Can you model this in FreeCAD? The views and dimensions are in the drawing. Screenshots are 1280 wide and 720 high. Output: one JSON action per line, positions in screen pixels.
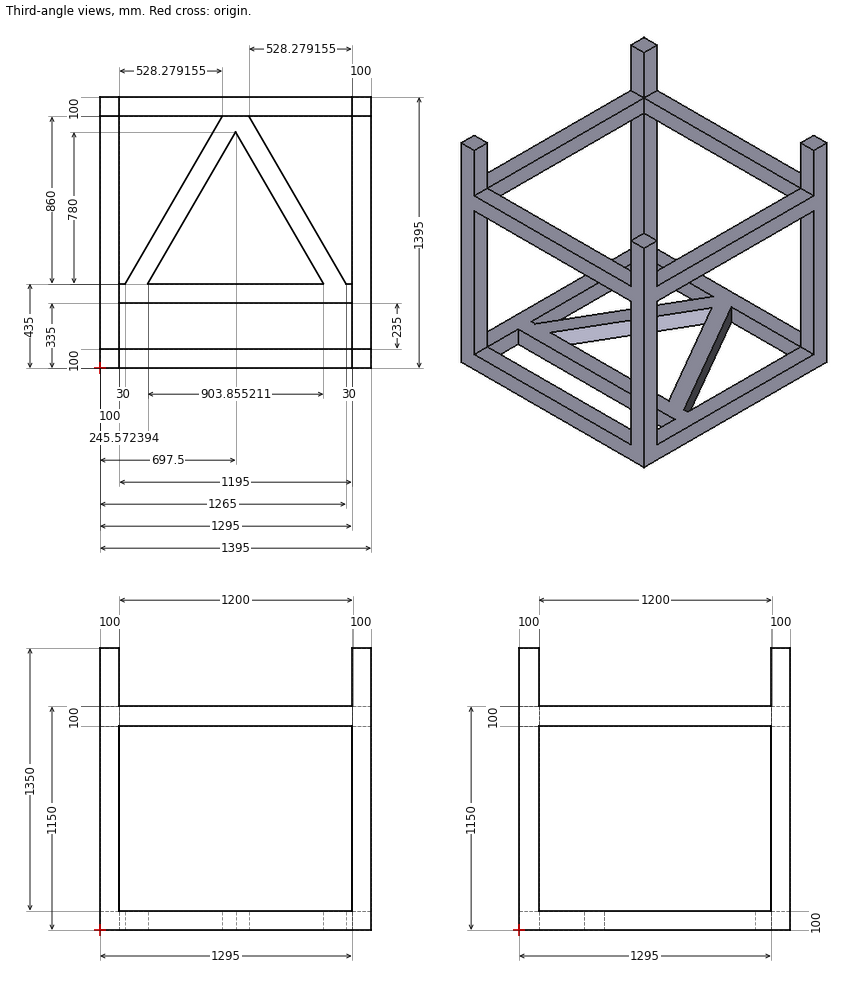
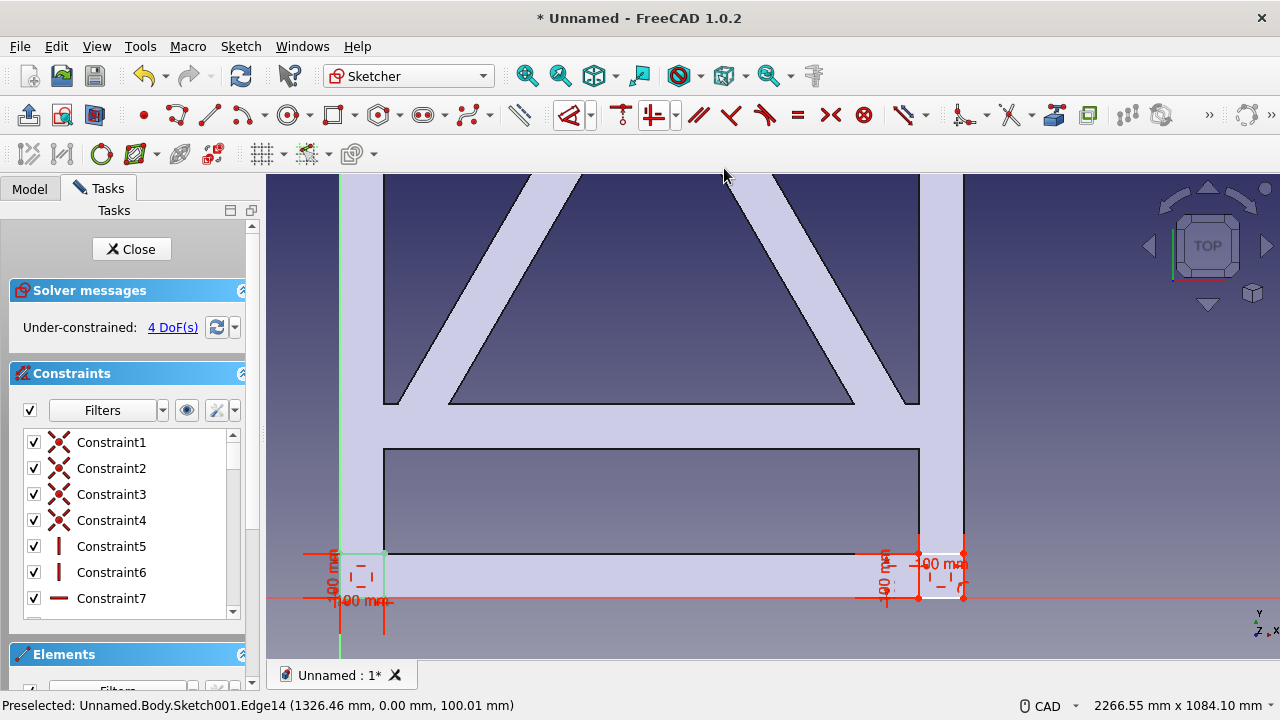
{"action": "scroll", "coordinate": [748, 523], "scroll_direction": "down", "scroll_amount": 4}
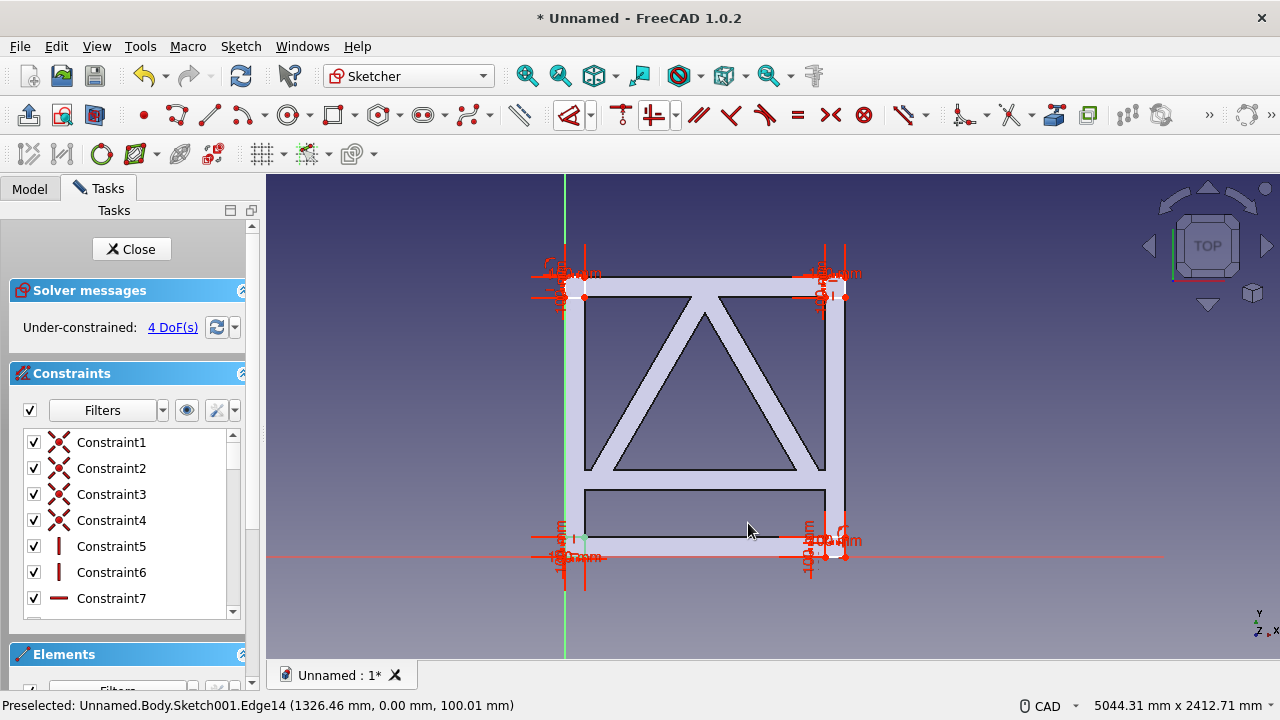
{"action": "left_click", "coordinate": [565, 277]}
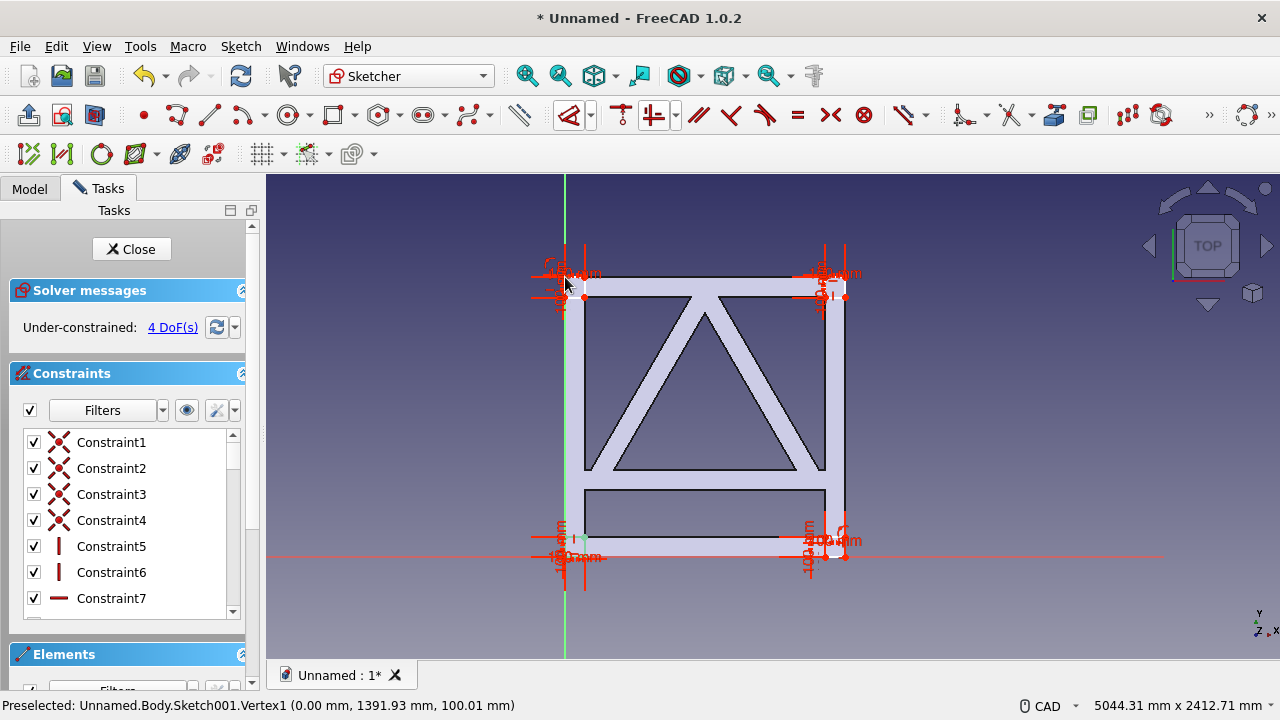
{"action": "left_click", "coordinate": [590, 116]}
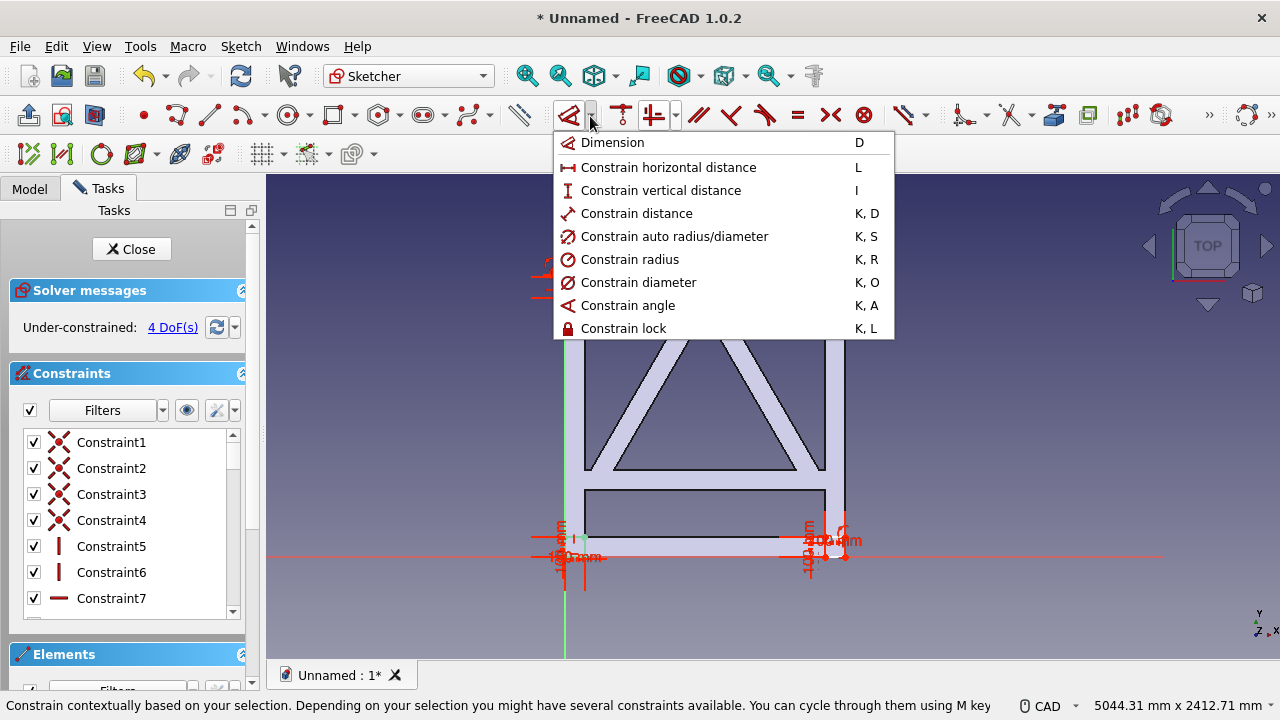
{"action": "left_click", "coordinate": [724, 190]}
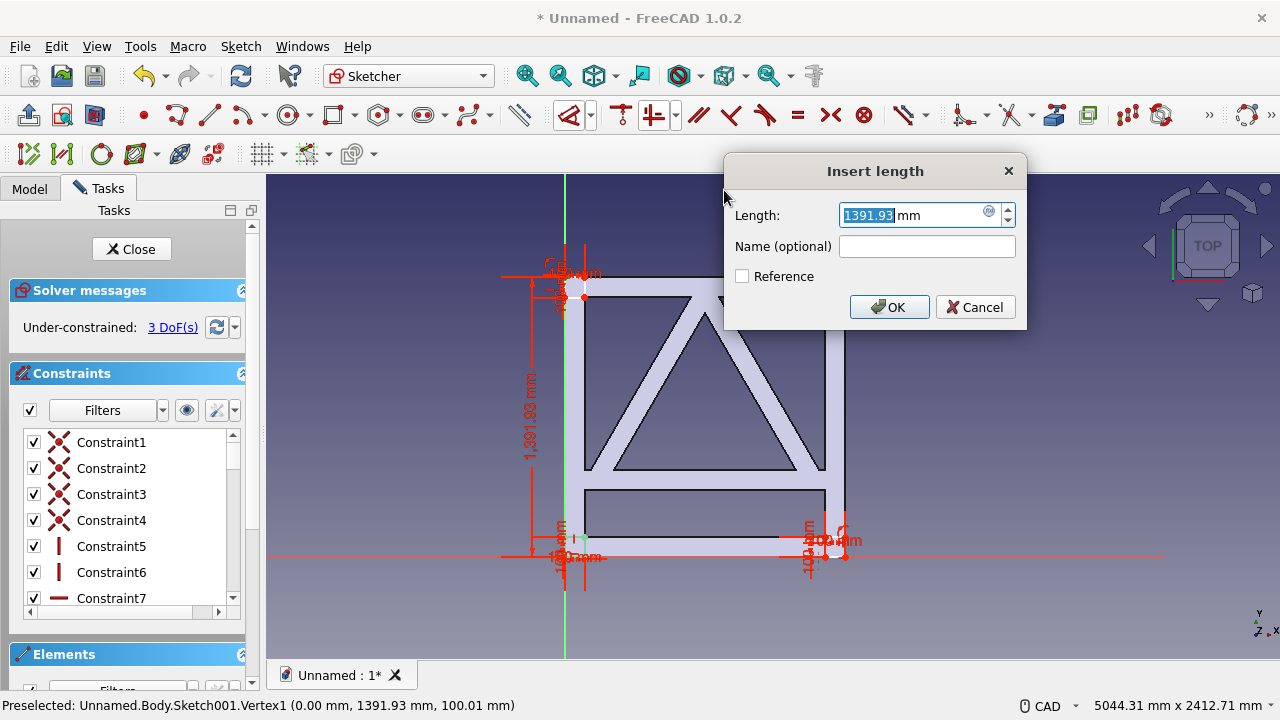
{"action": "type", "text": "1395"}
{"action": "key", "text": "Return"}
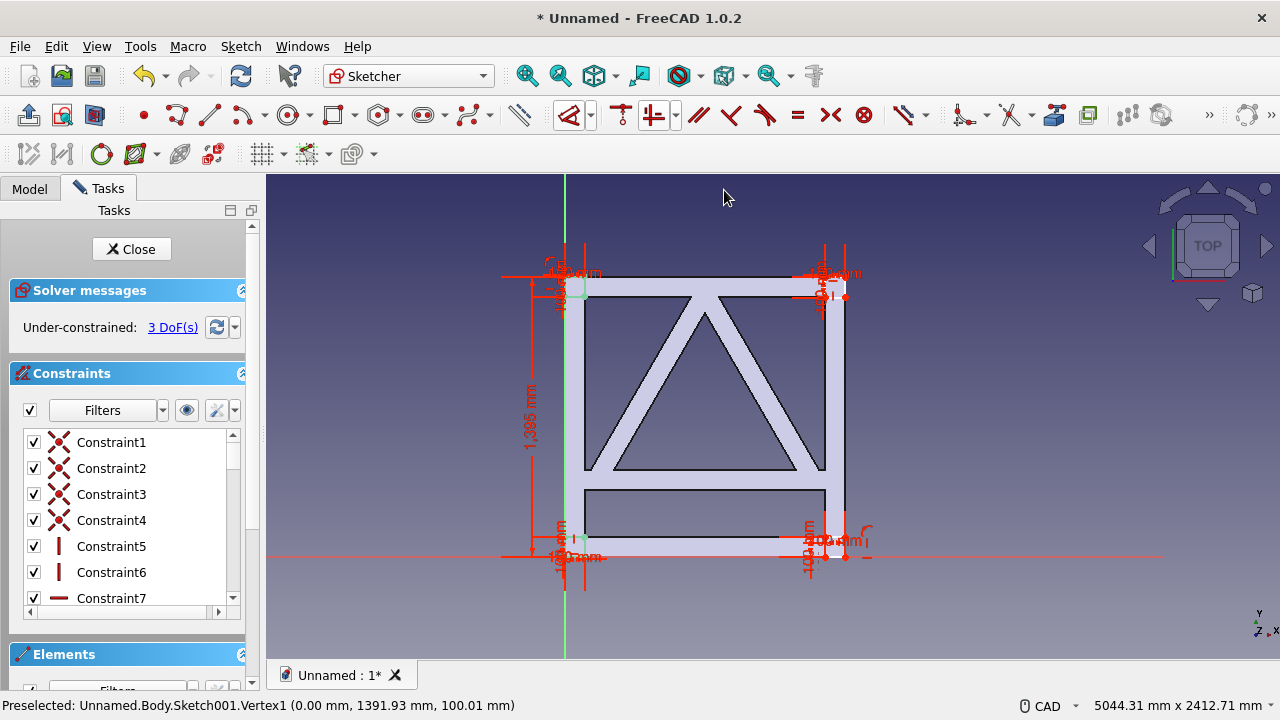
{"action": "left_click", "coordinate": [825, 277]}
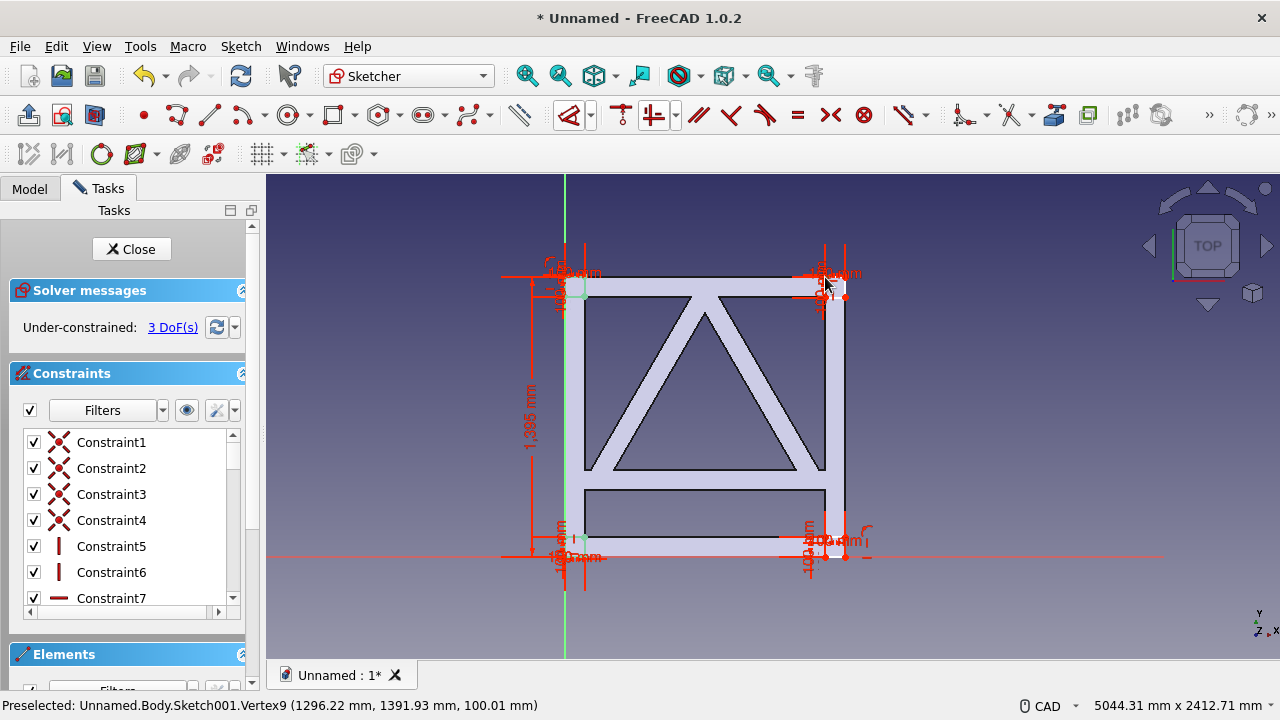
{"action": "left_click", "coordinate": [590, 116]}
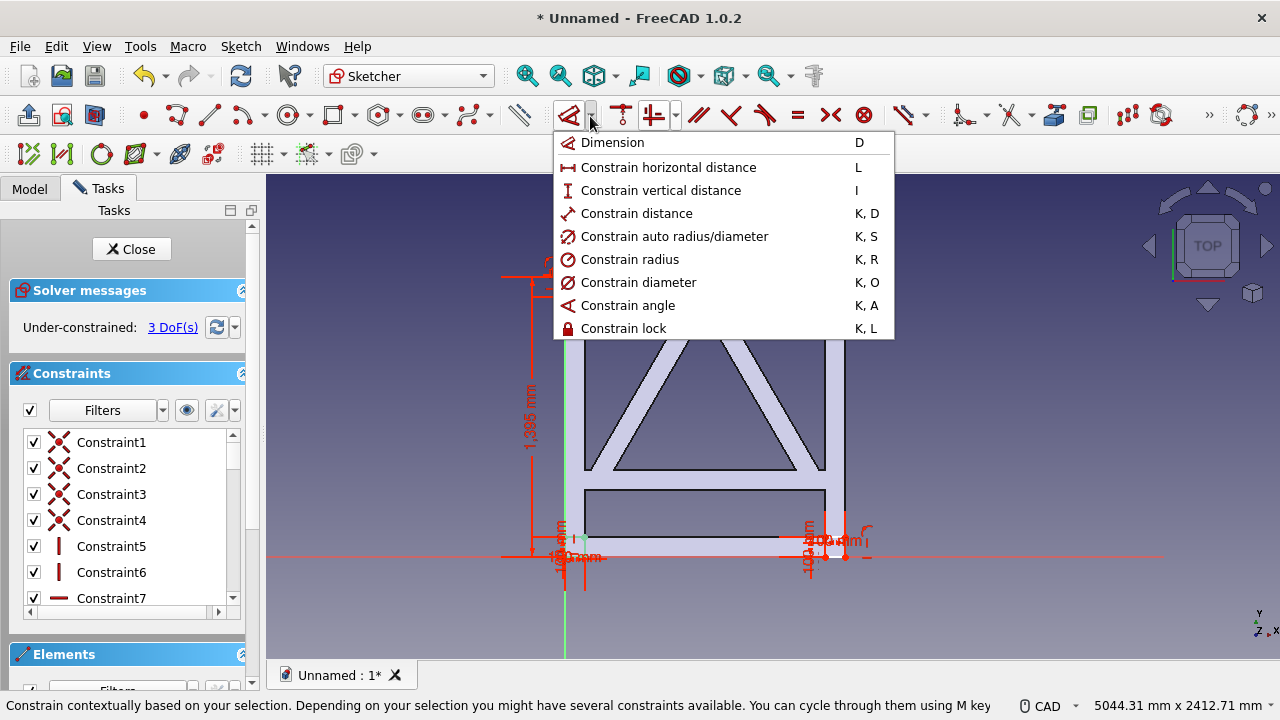
{"action": "left_click", "coordinate": [724, 168]}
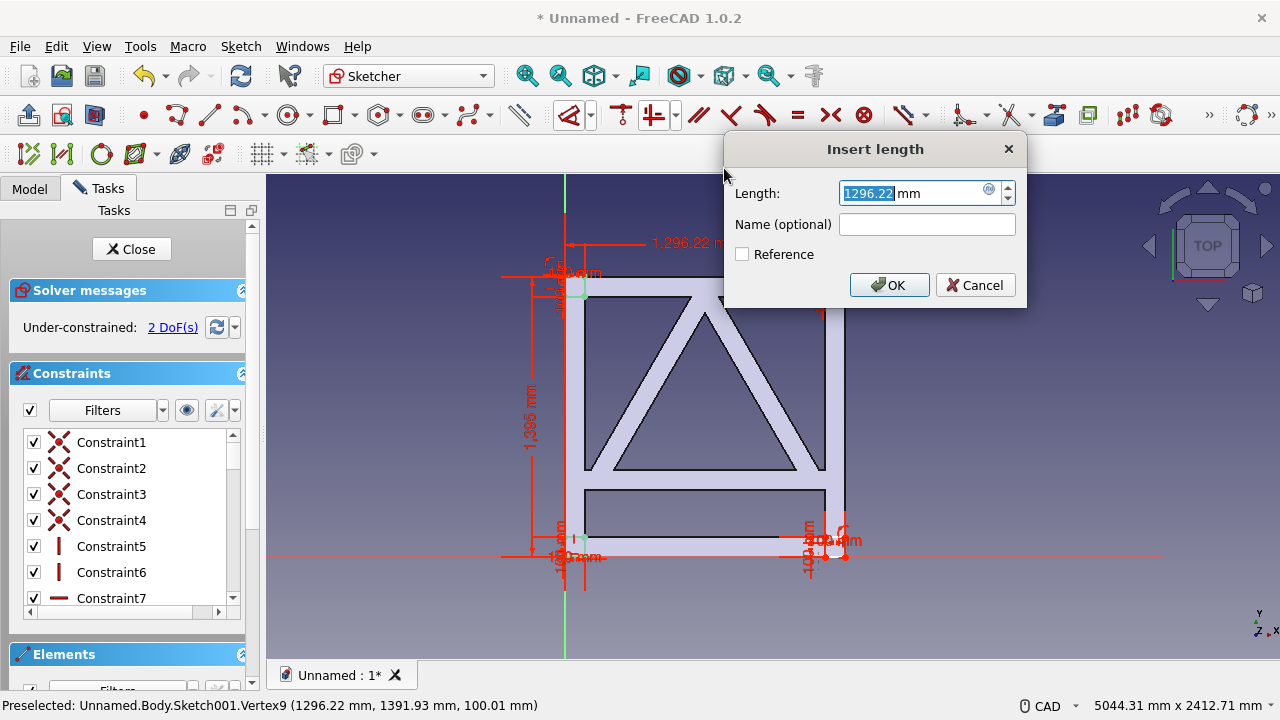
{"action": "type", "text": "1295"}
{"action": "key", "text": "Return"}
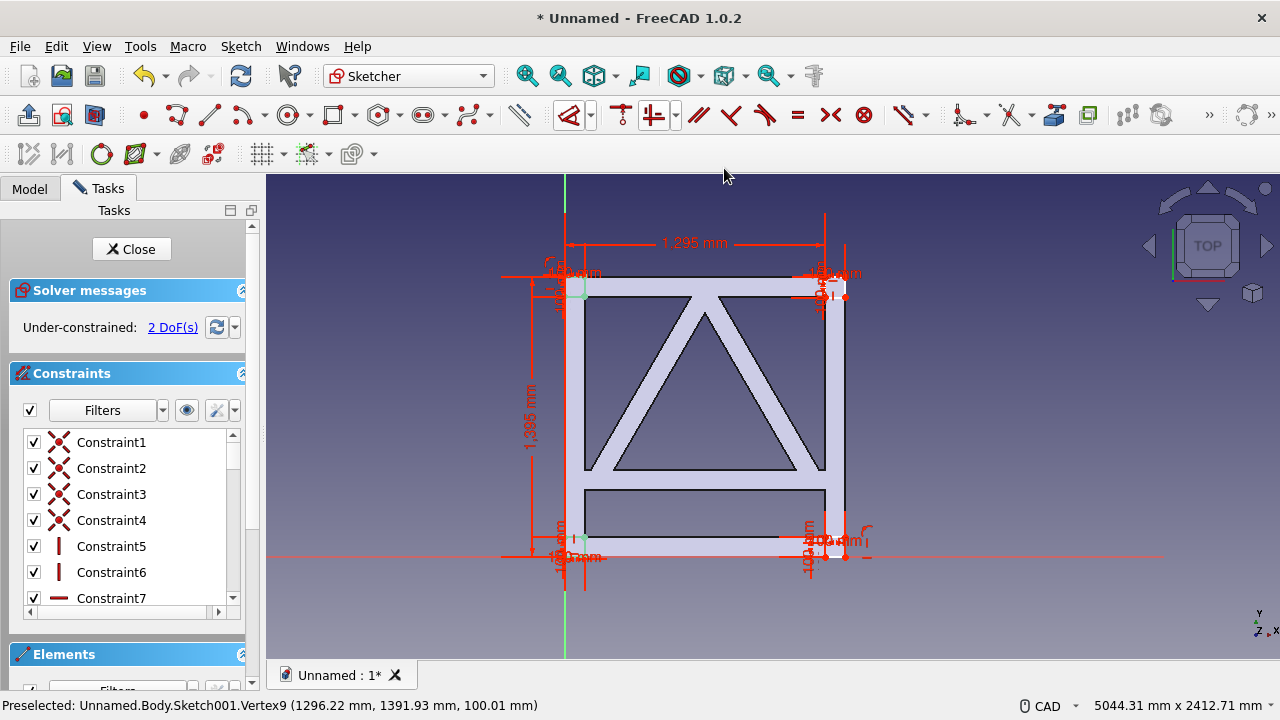
{"action": "left_click", "coordinate": [825, 277]}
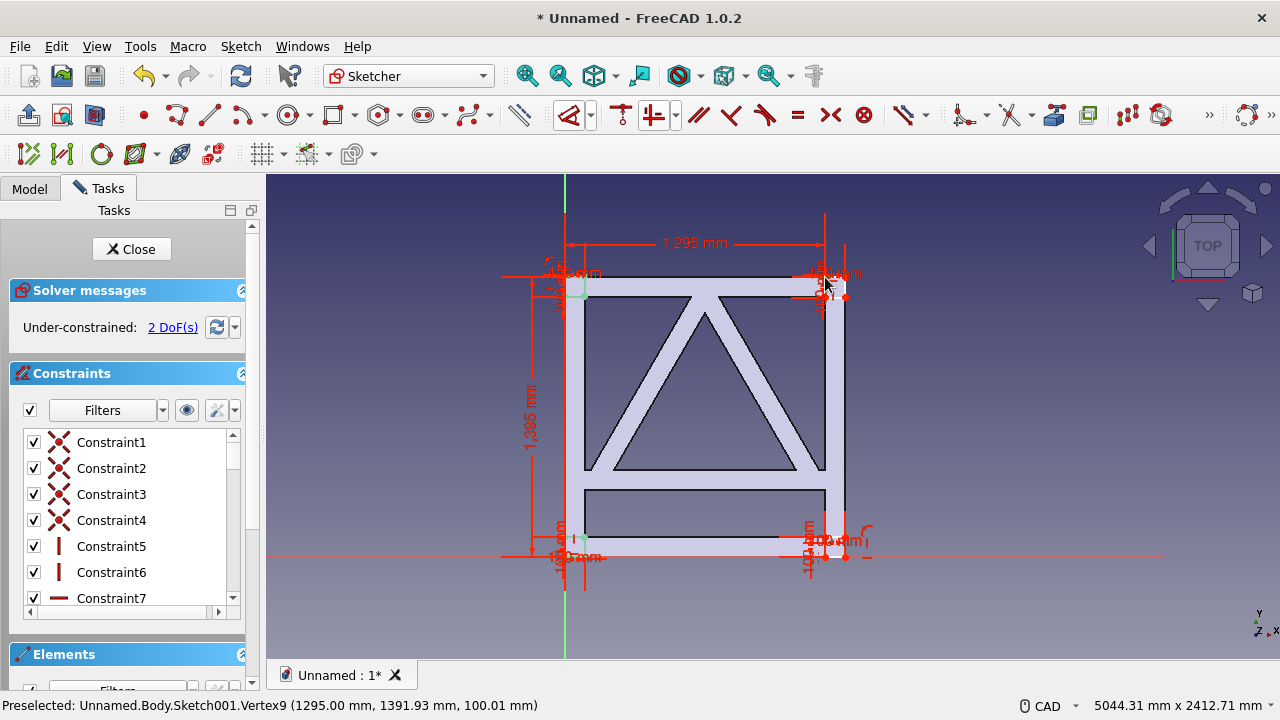
{"action": "left_click", "coordinate": [590, 116]}